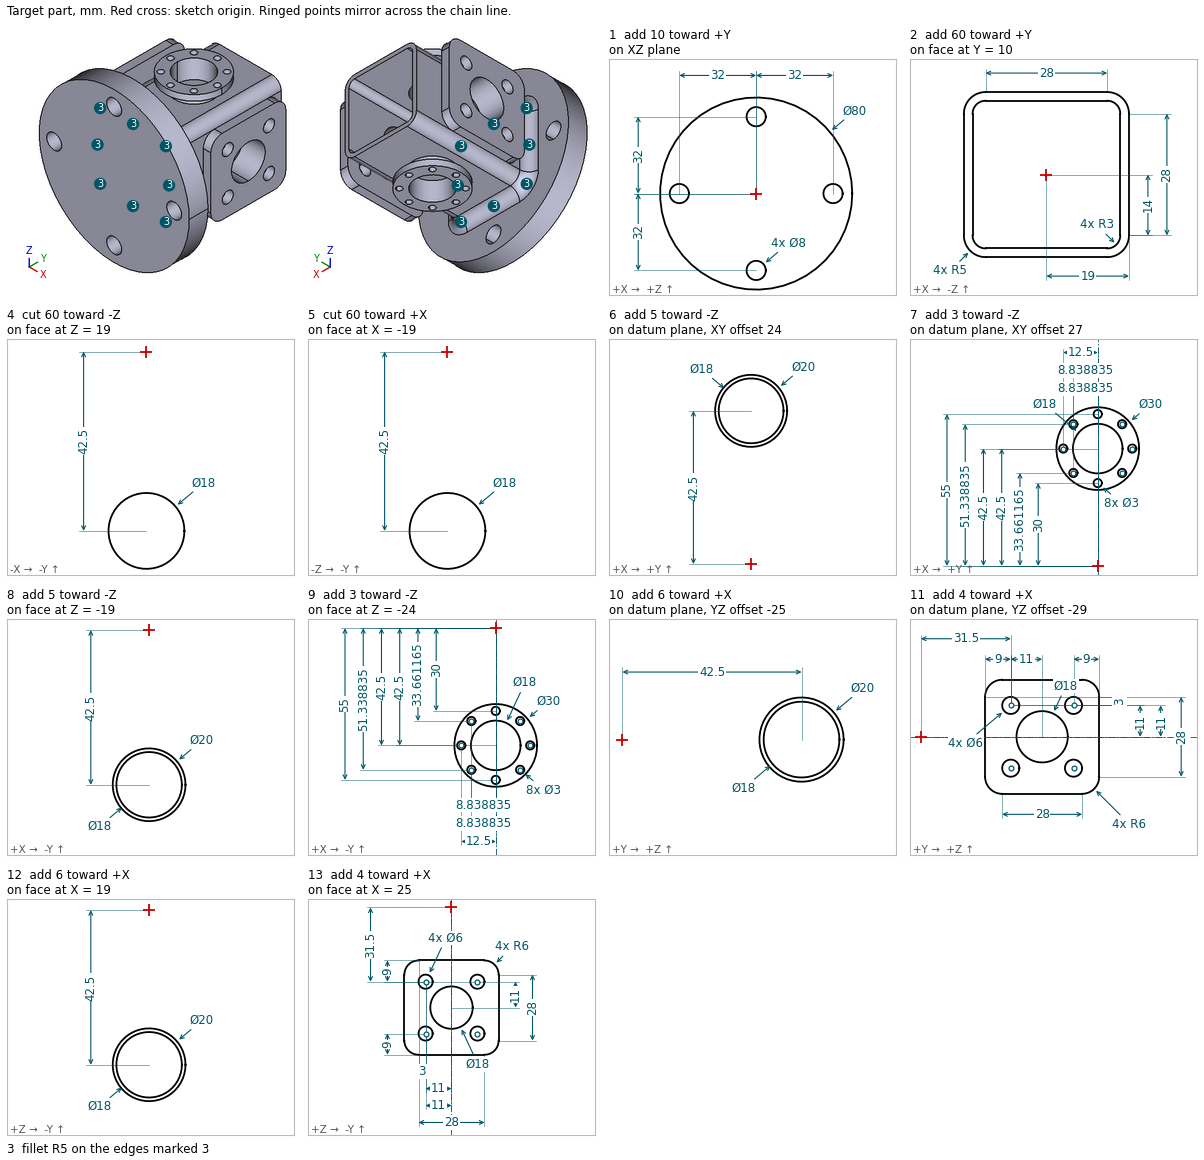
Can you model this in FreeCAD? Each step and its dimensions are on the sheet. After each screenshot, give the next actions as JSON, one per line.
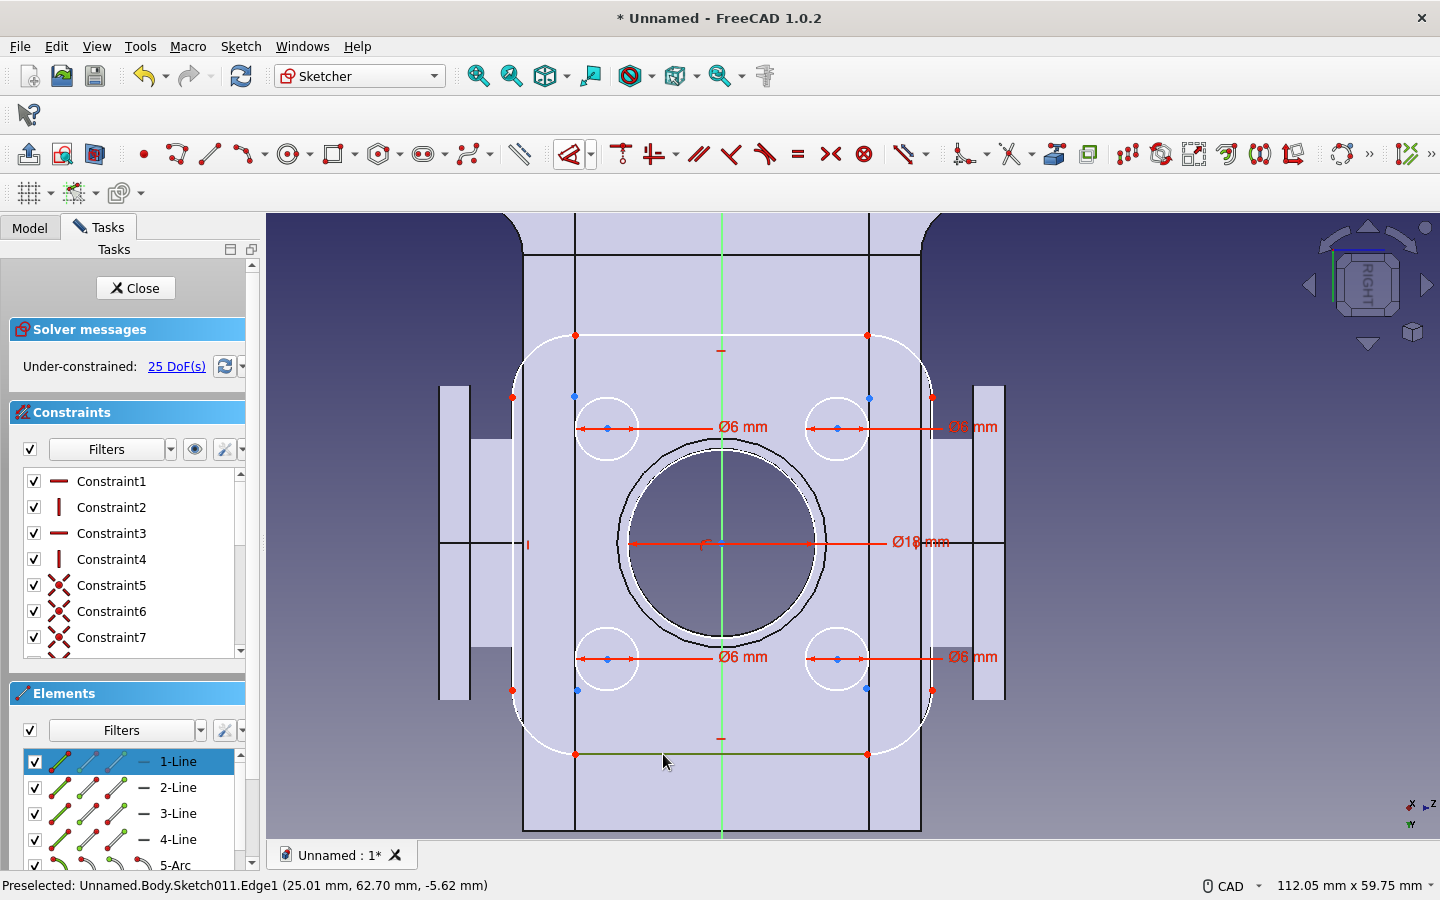
{"action": "left_click", "coordinate": [897, 747]}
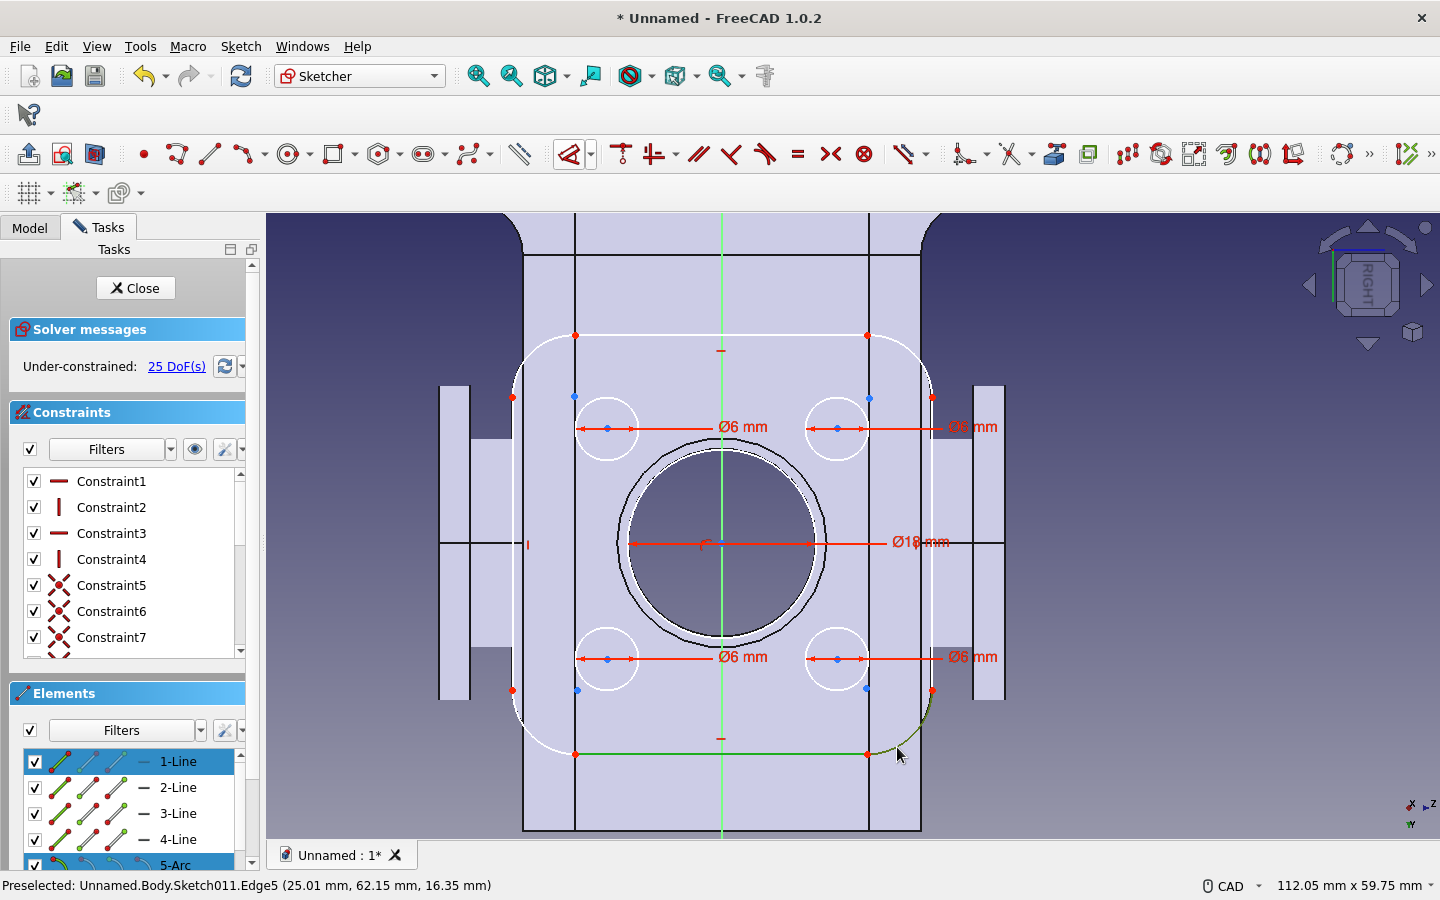
{"action": "key", "text": "t"}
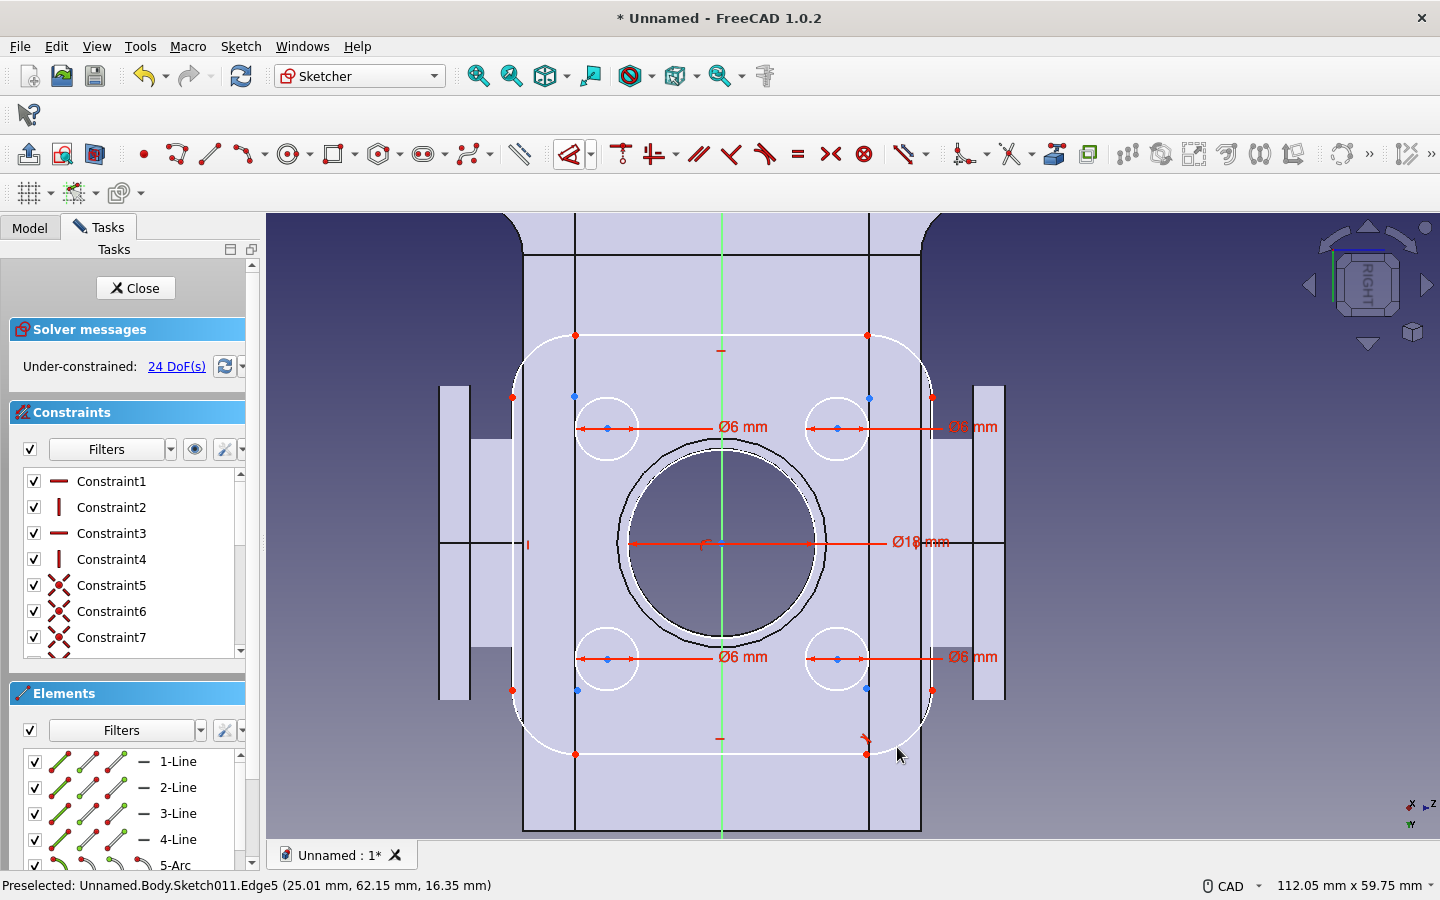
{"action": "left_click", "coordinate": [663, 754]}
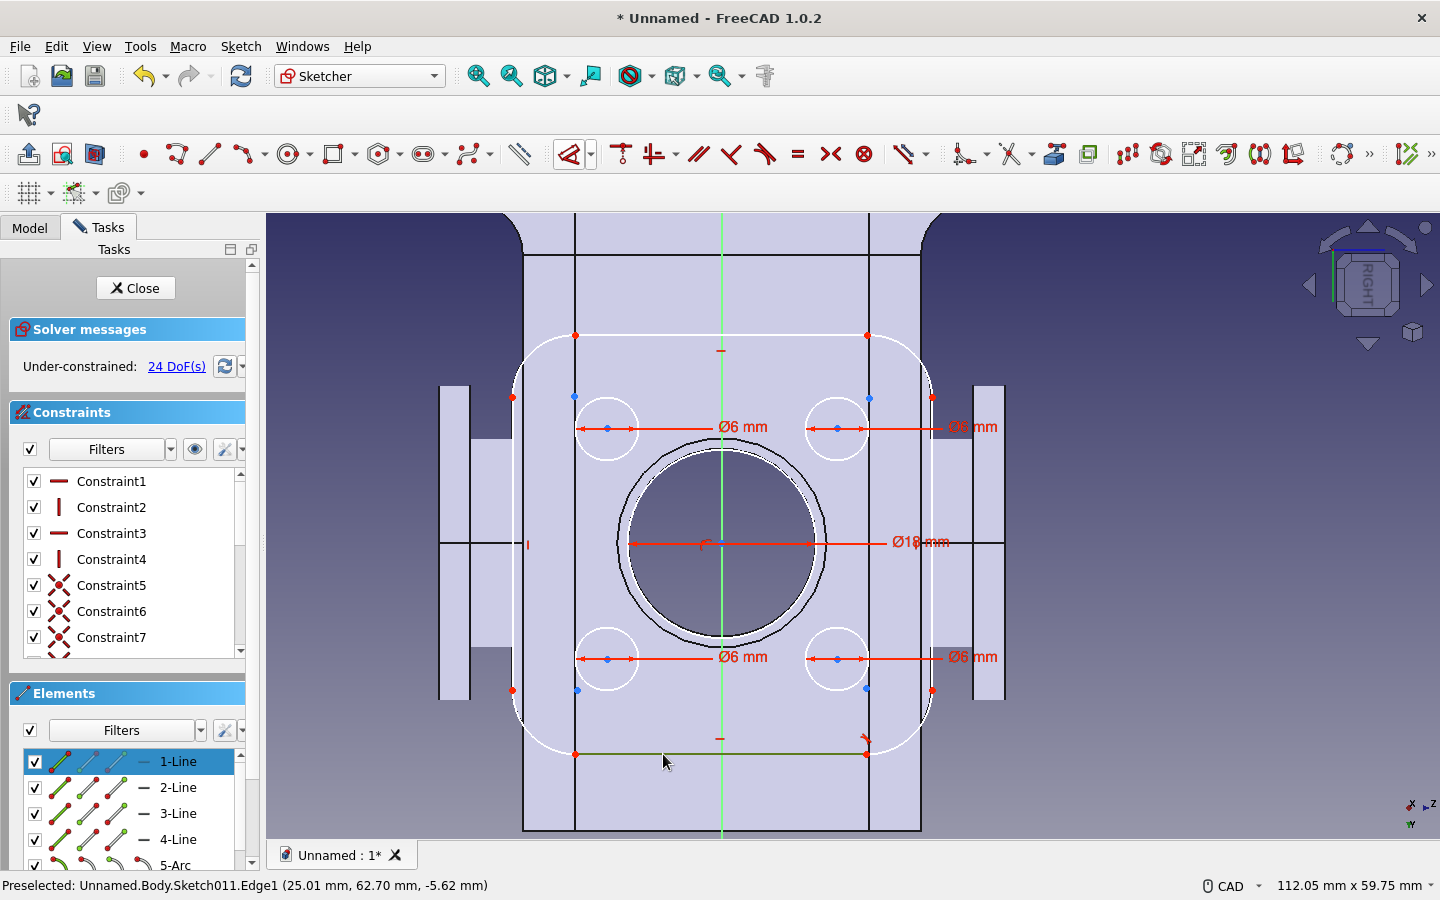
{"action": "left_click", "coordinate": [520, 719]}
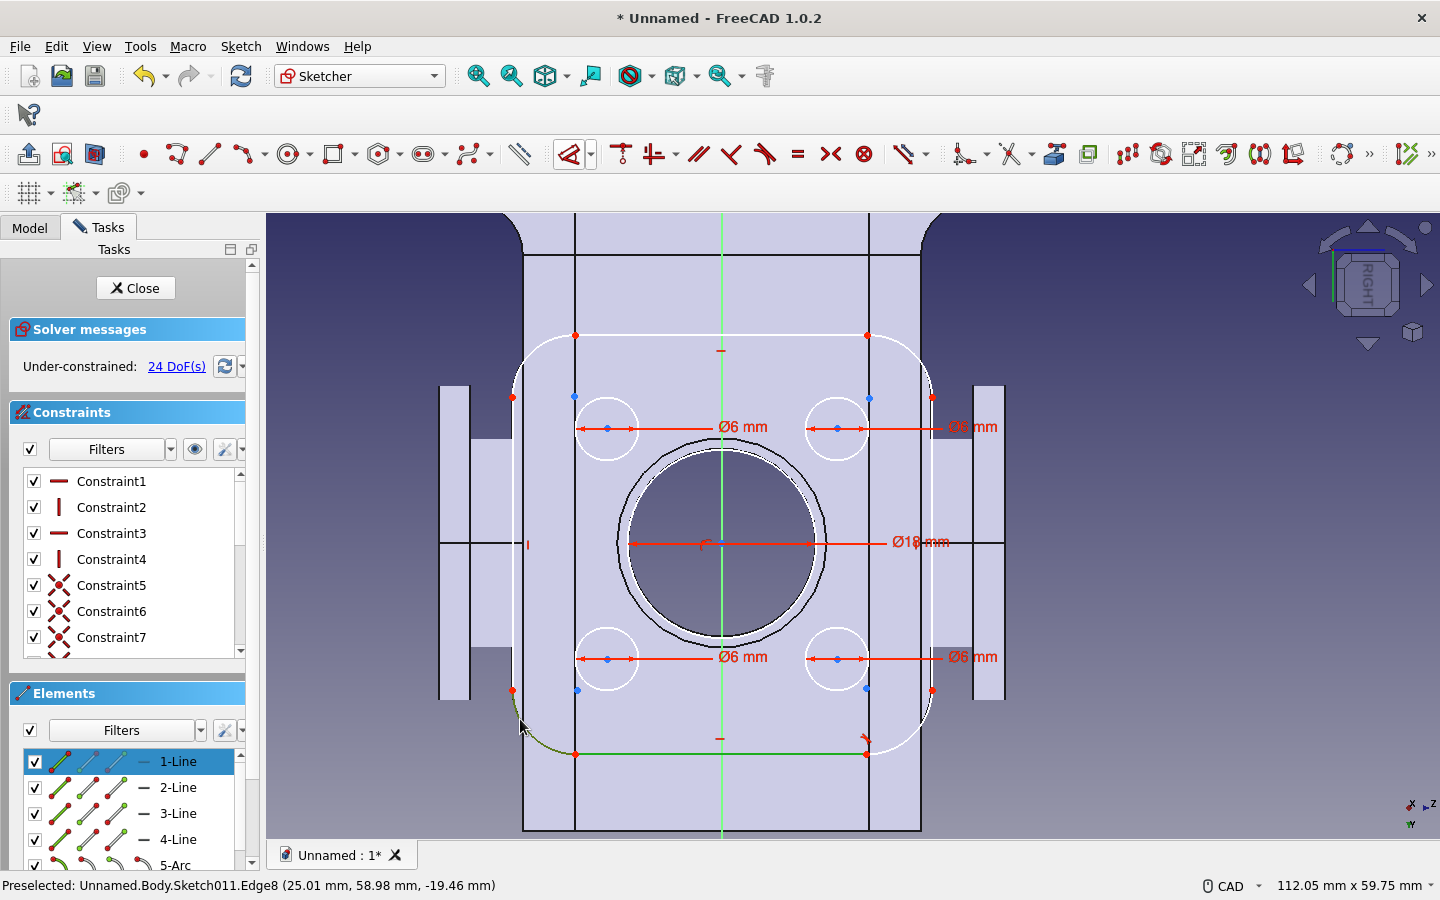
{"action": "key", "text": "t"}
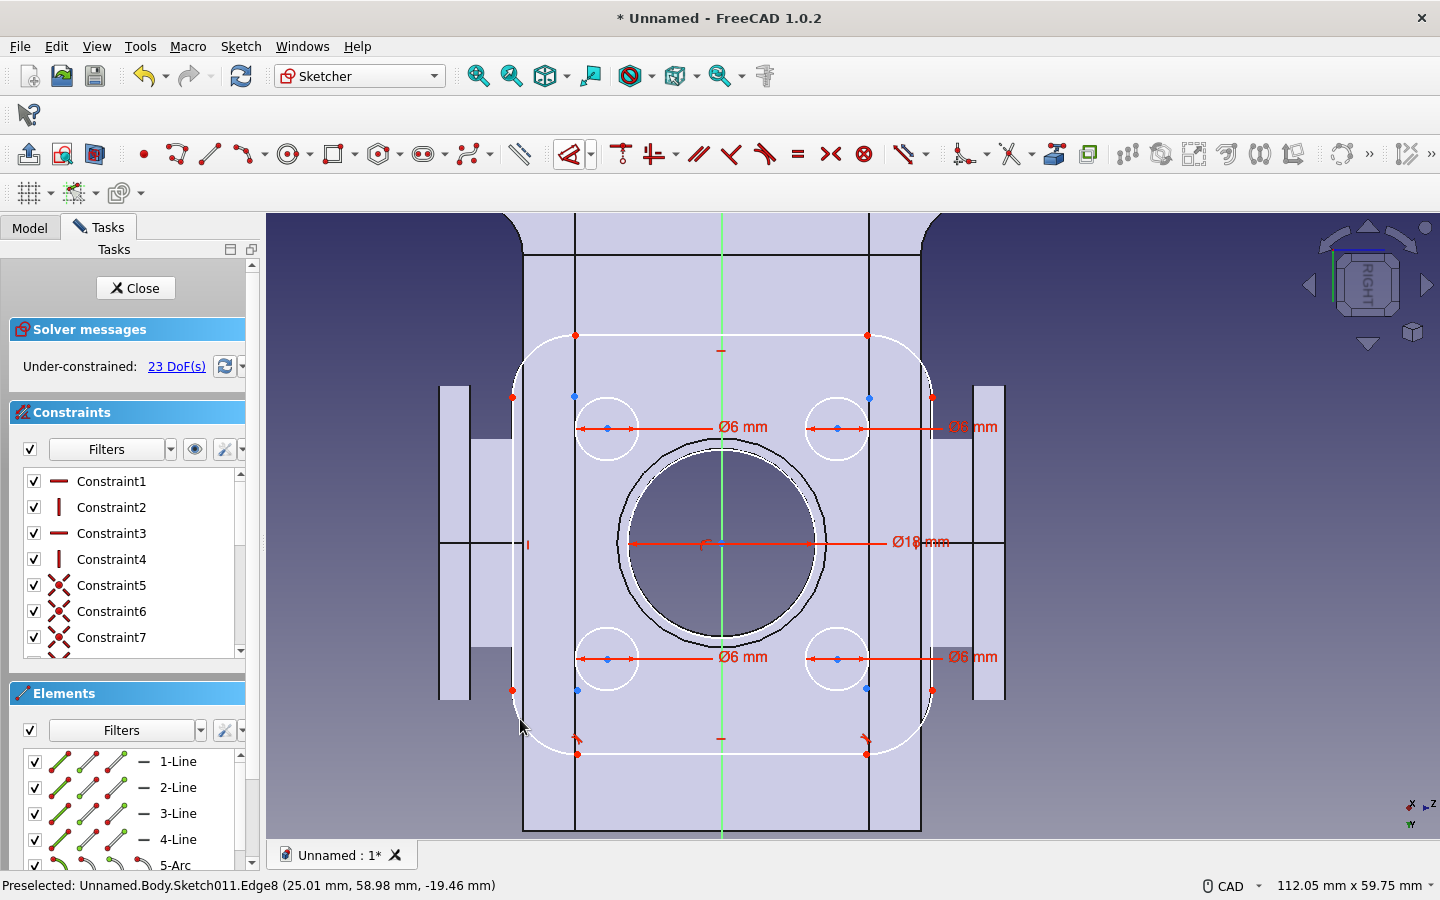
{"action": "left_click", "coordinate": [932, 603]}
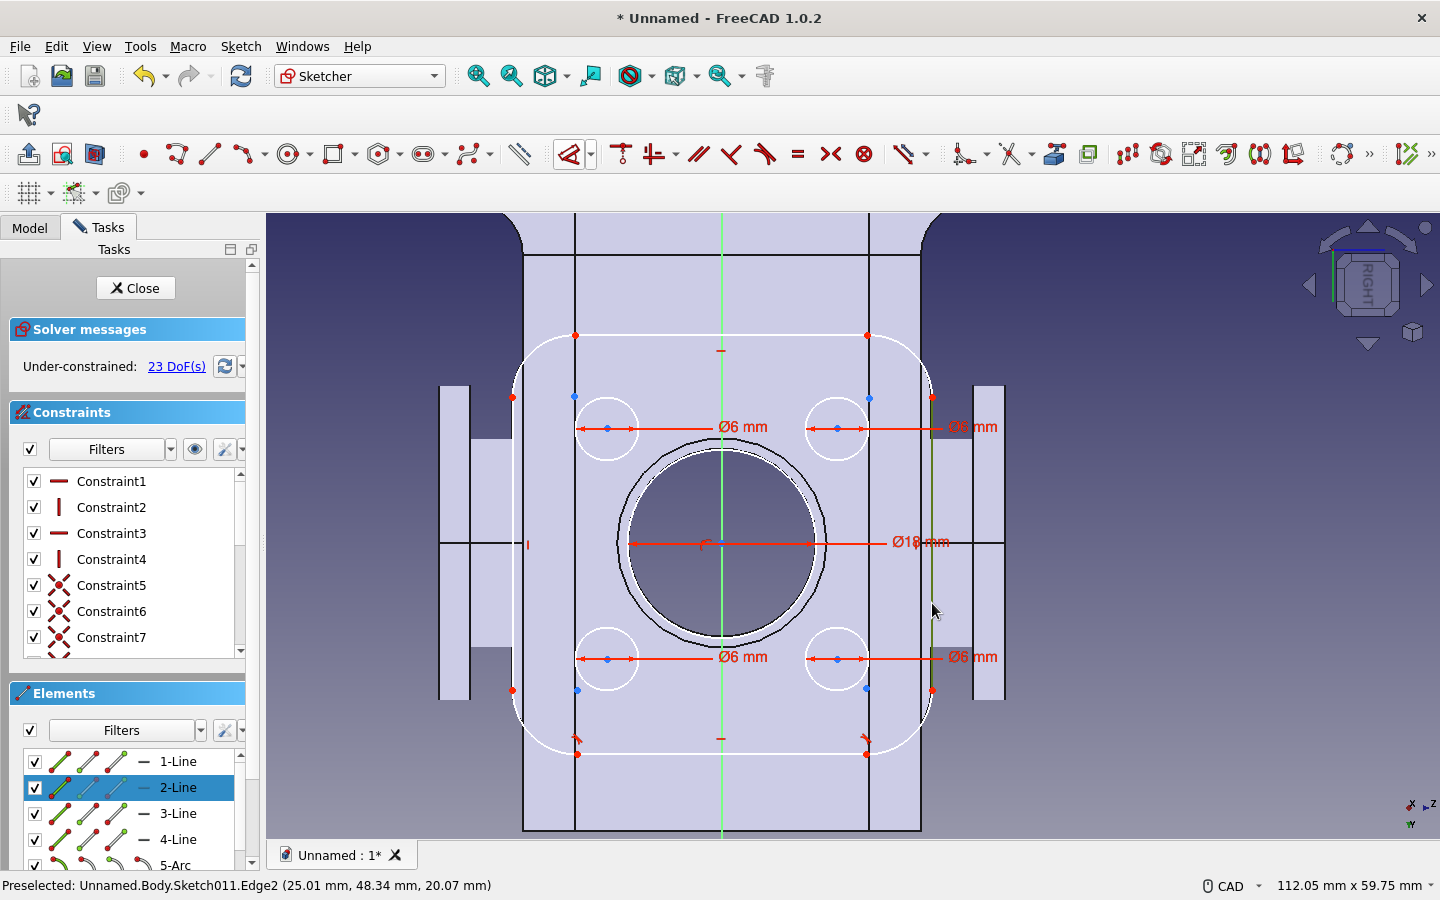
{"action": "left_click", "coordinate": [896, 748]}